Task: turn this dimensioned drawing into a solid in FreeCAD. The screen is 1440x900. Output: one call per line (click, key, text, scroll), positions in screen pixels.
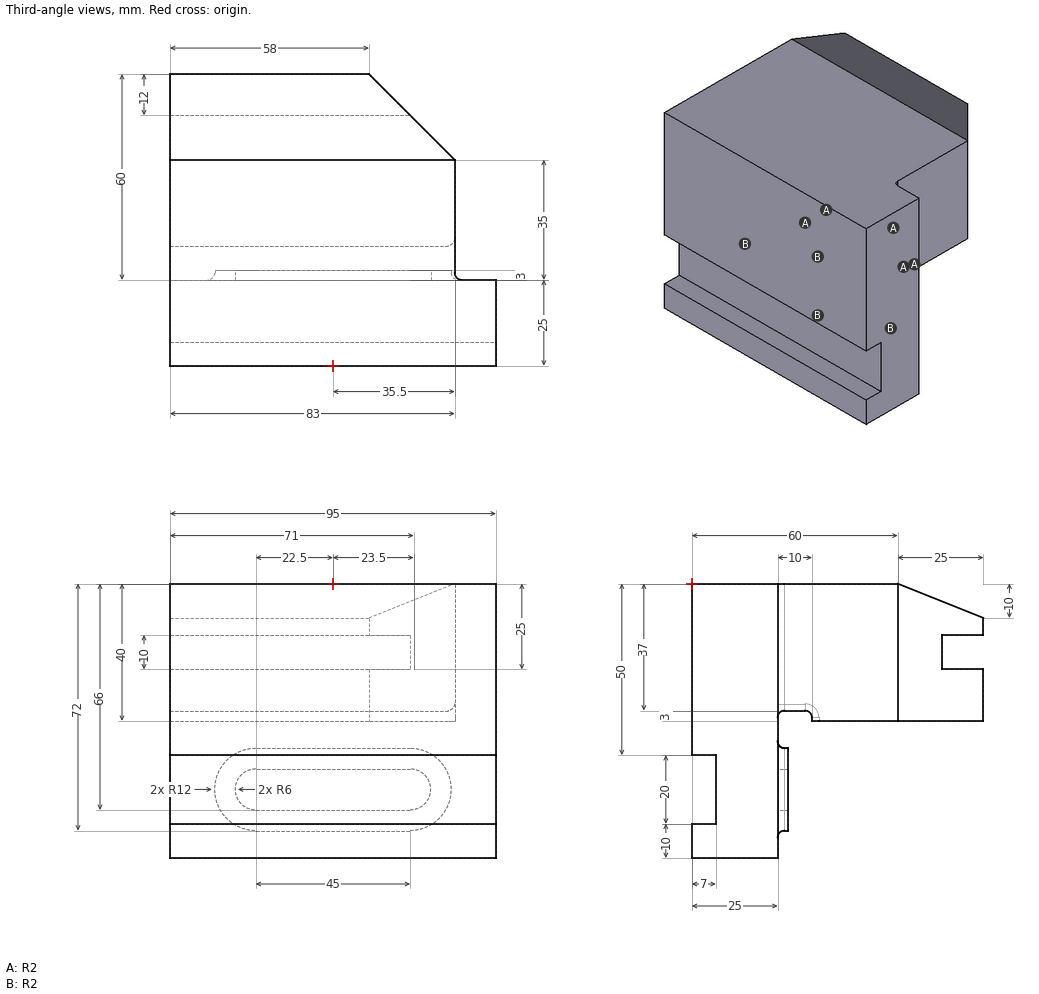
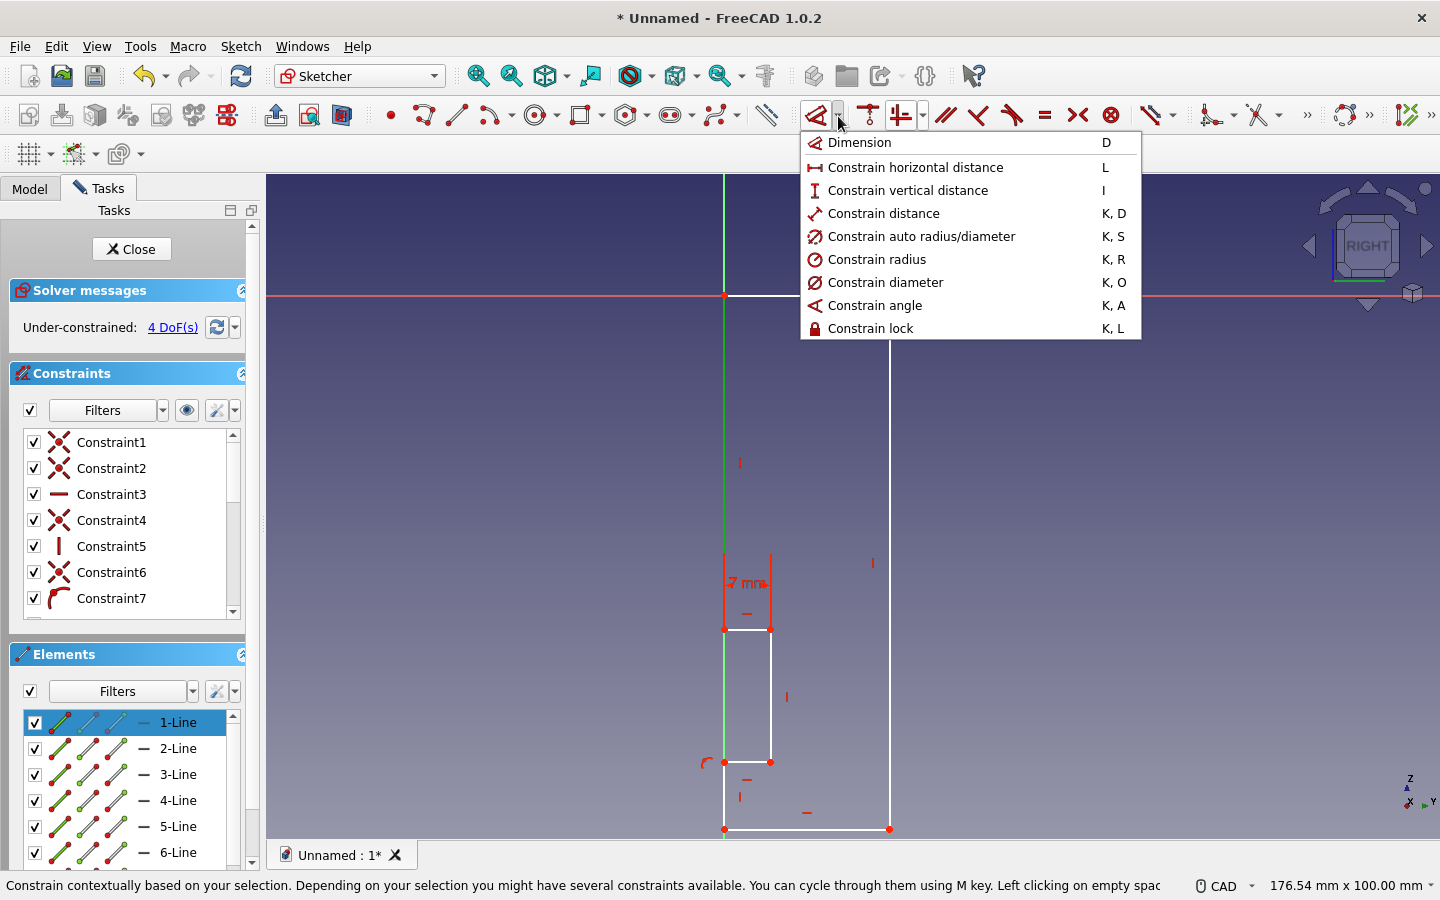
click(971, 190)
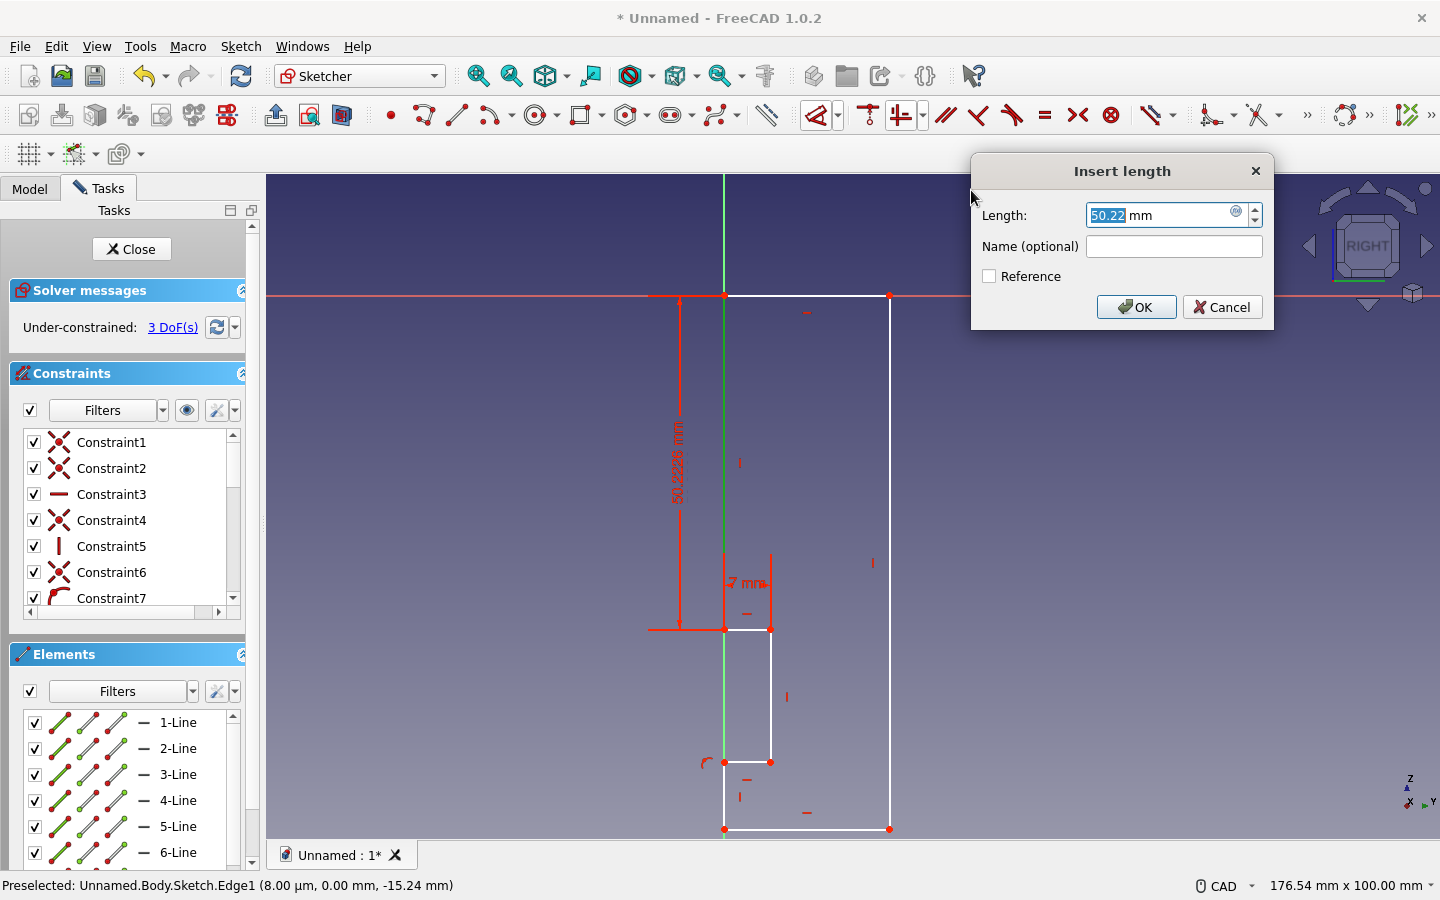
text(50)
key(Return)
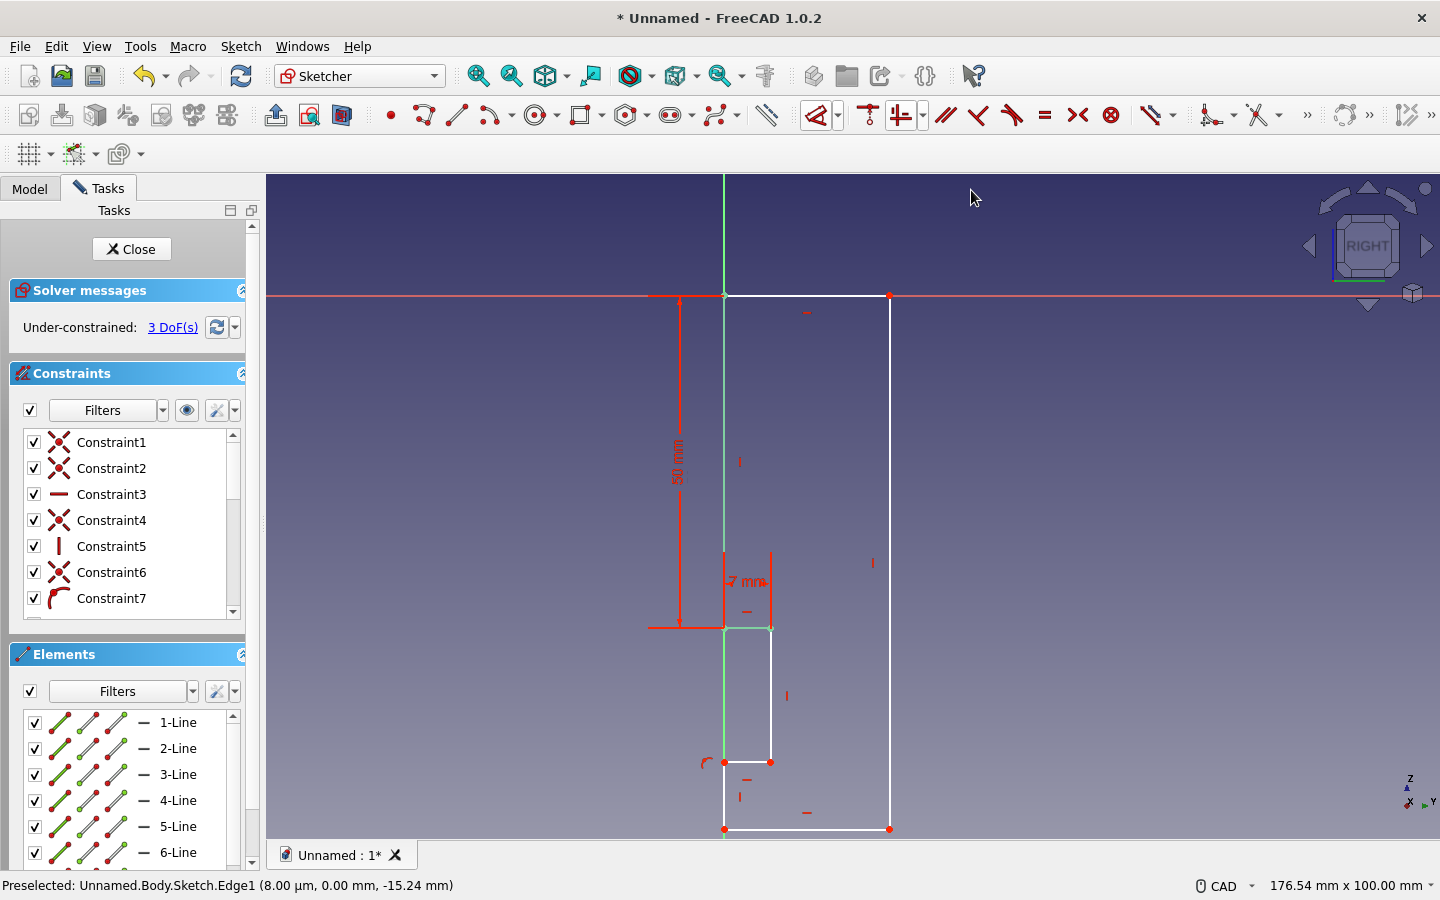
click(771, 668)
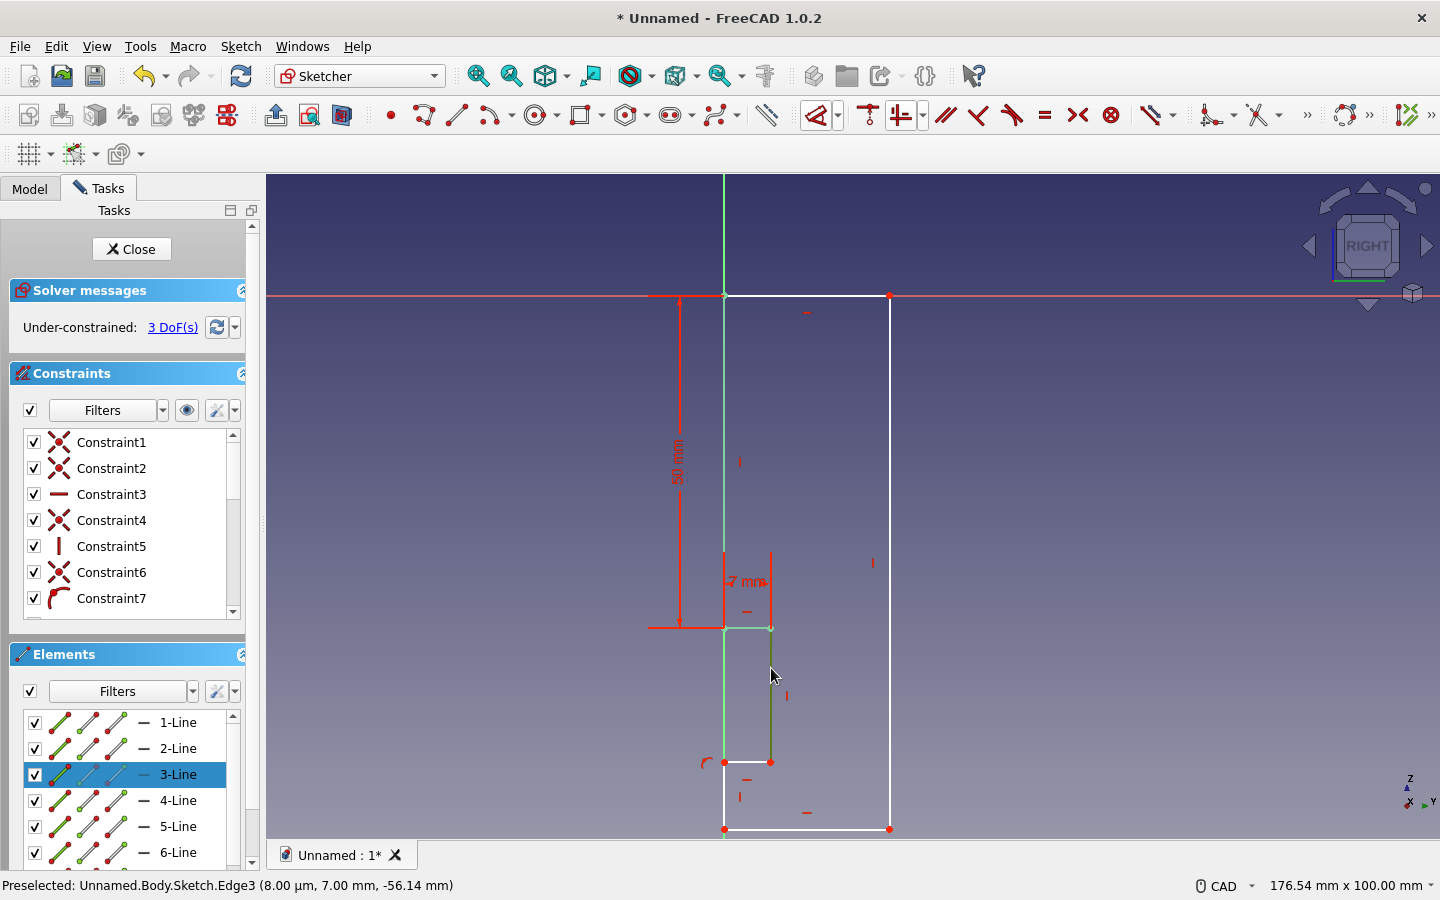
key(i)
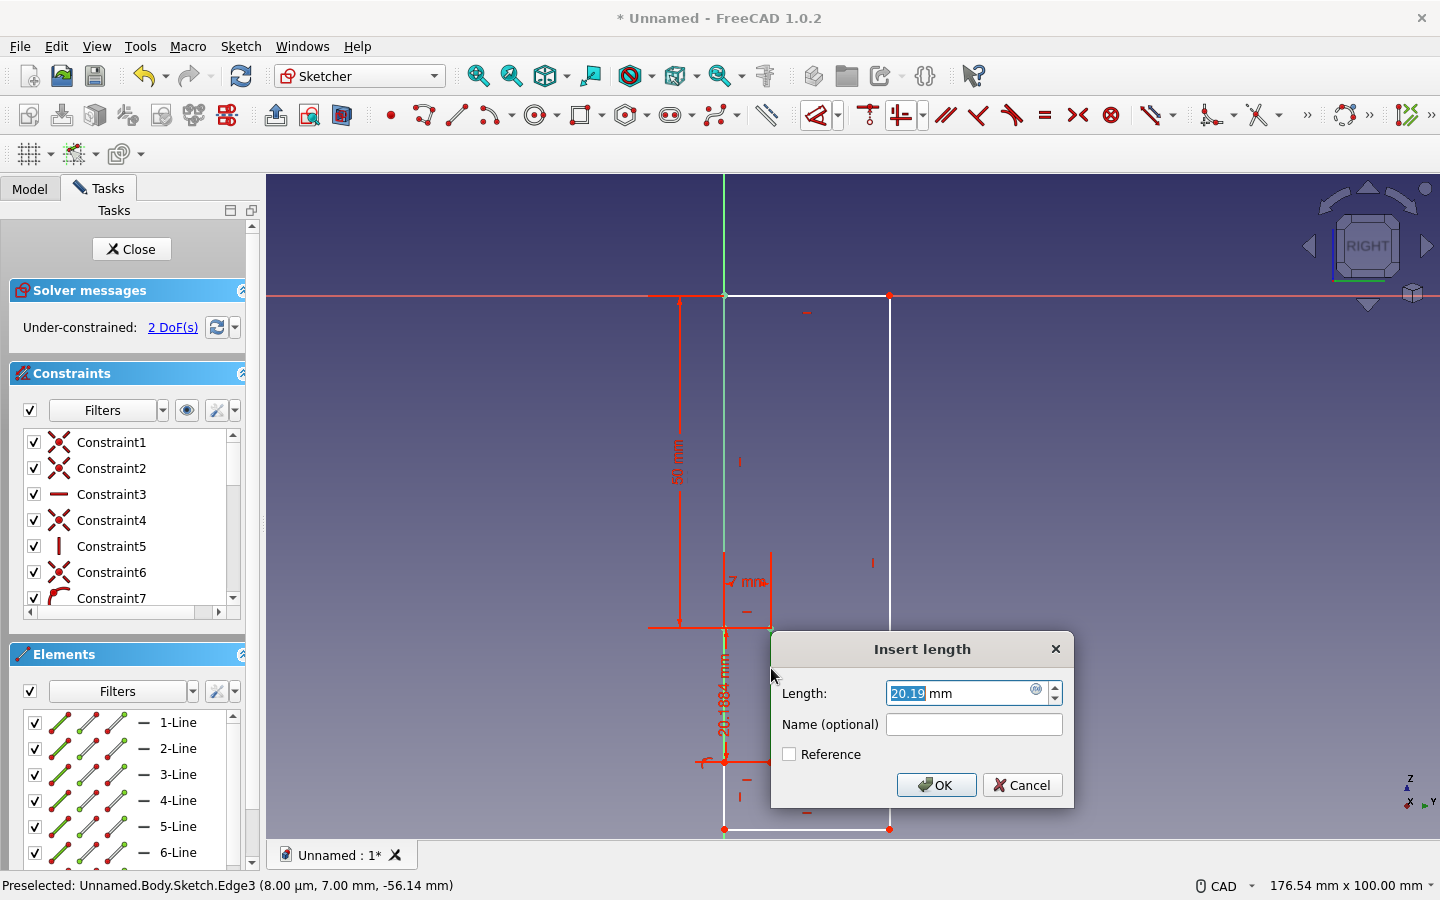
text(20)
key(Return)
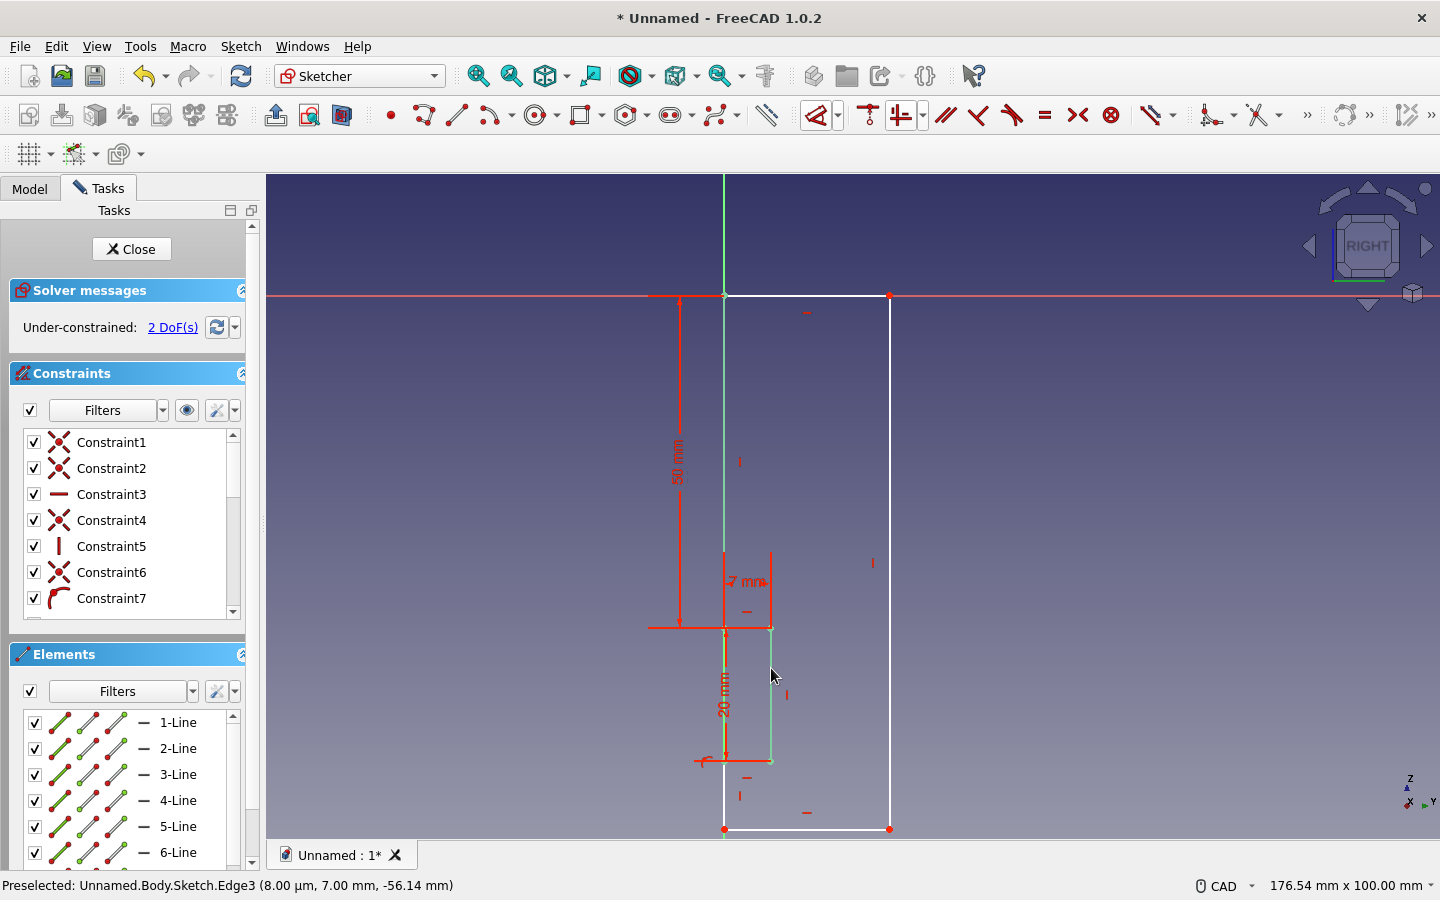
click(724, 782)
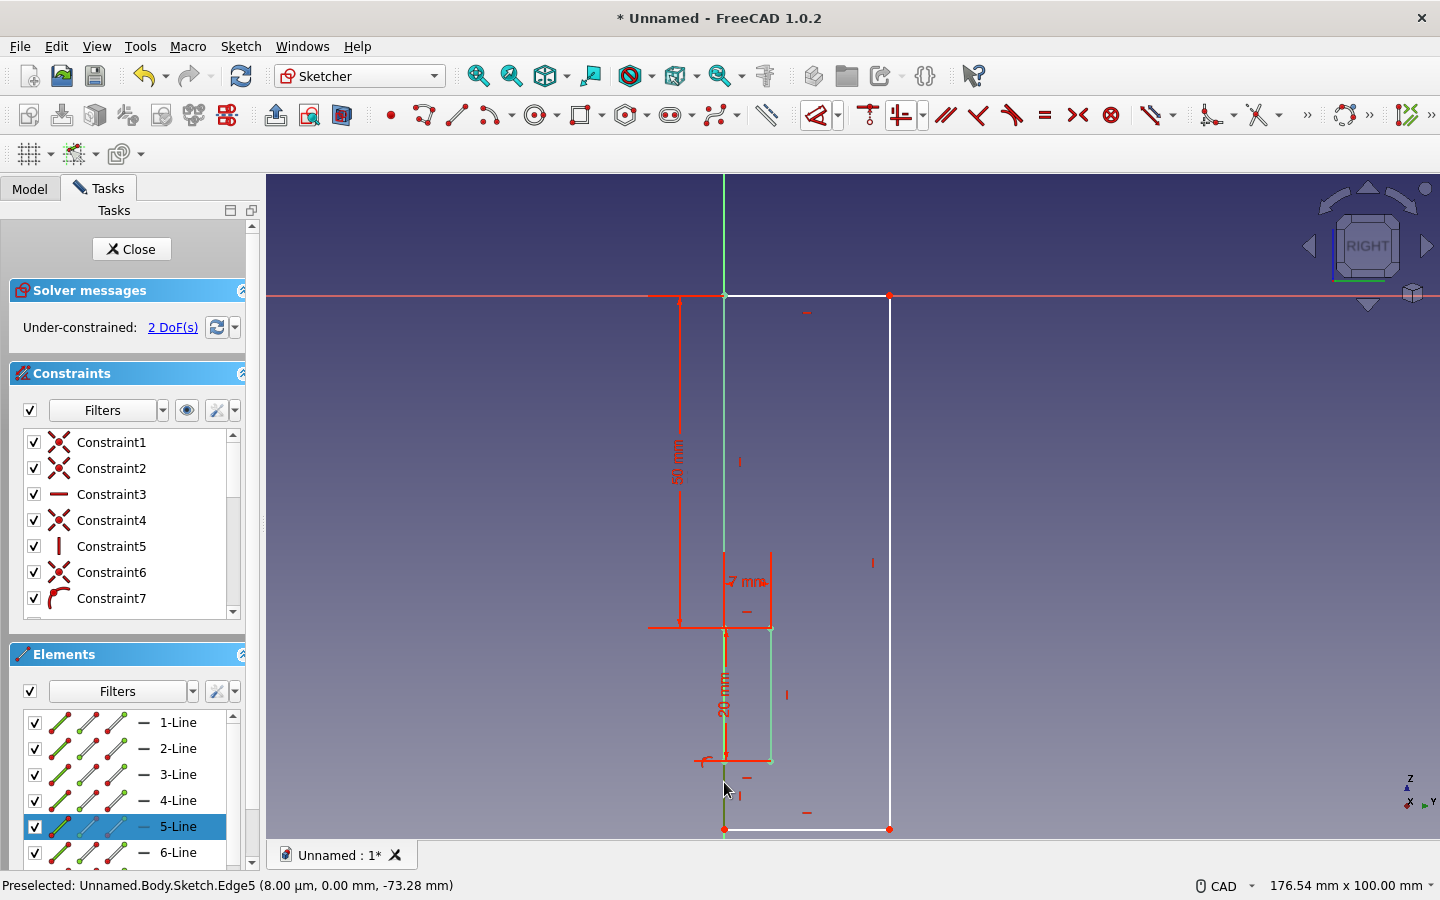
click(838, 116)